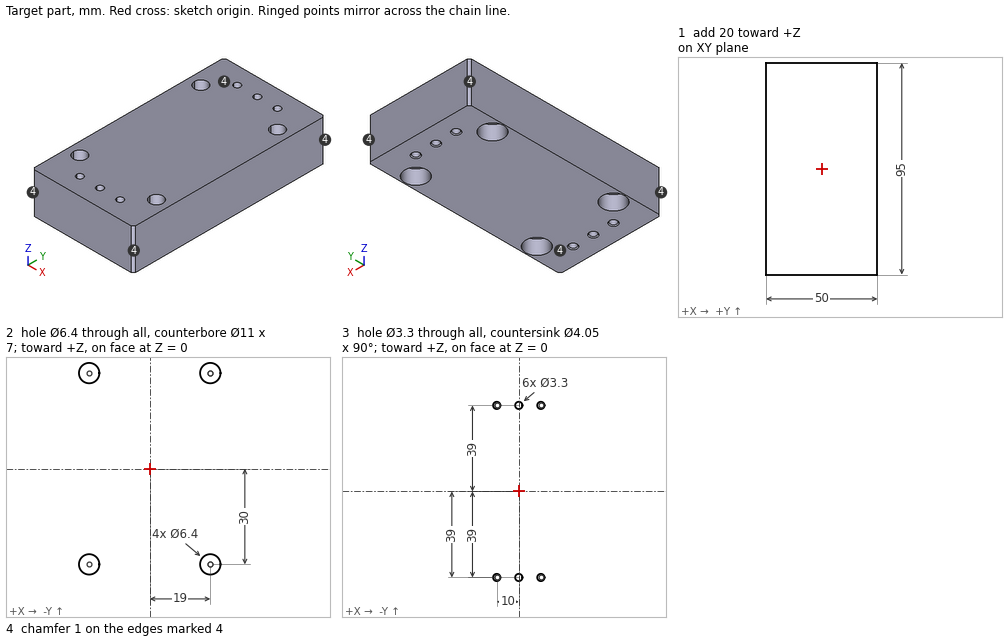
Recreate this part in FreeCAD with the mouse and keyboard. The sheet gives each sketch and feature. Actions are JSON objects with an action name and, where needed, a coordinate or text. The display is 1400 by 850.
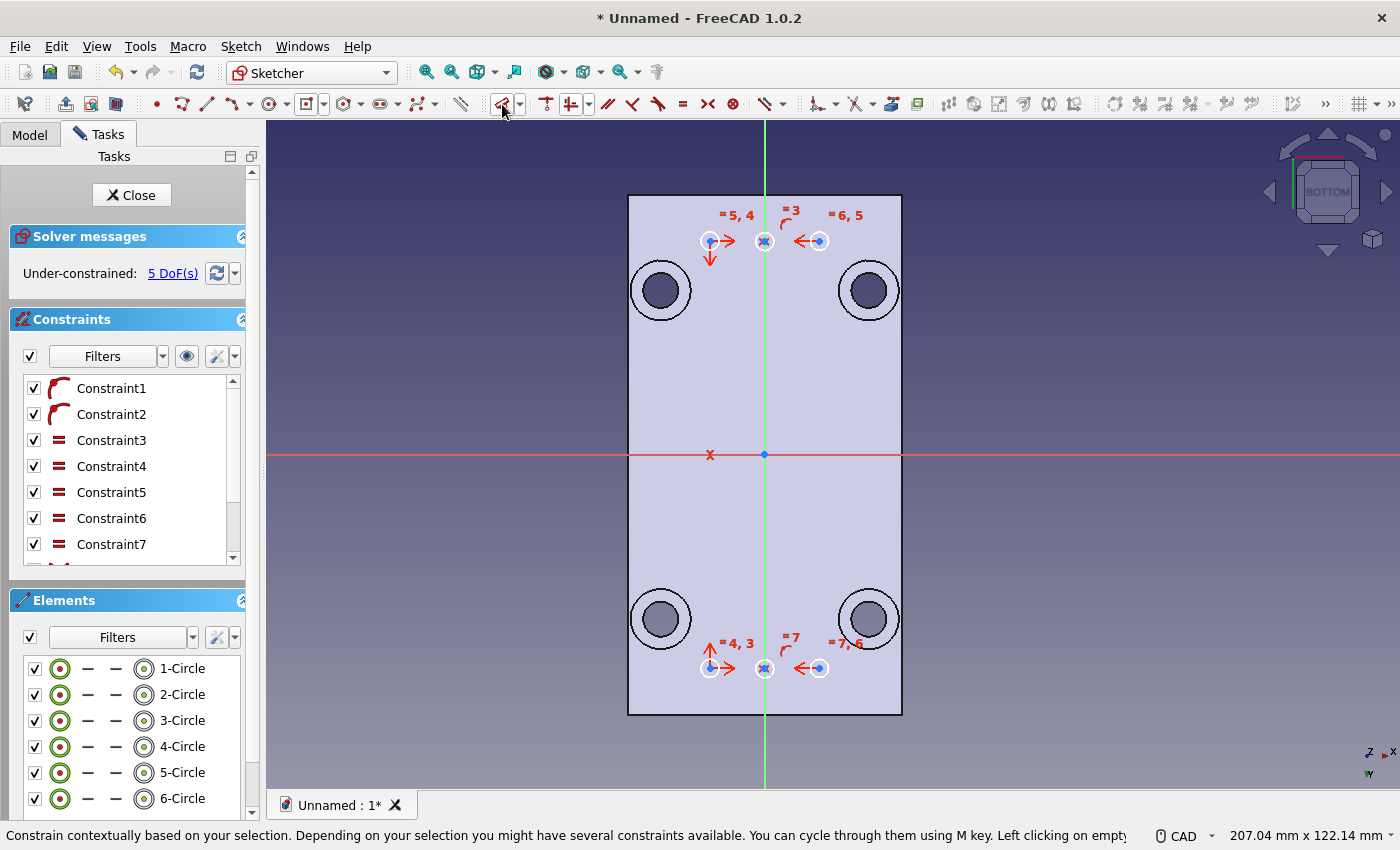
{"action": "scroll", "coordinate": [765, 233], "scroll_direction": "up", "scroll_amount": 4}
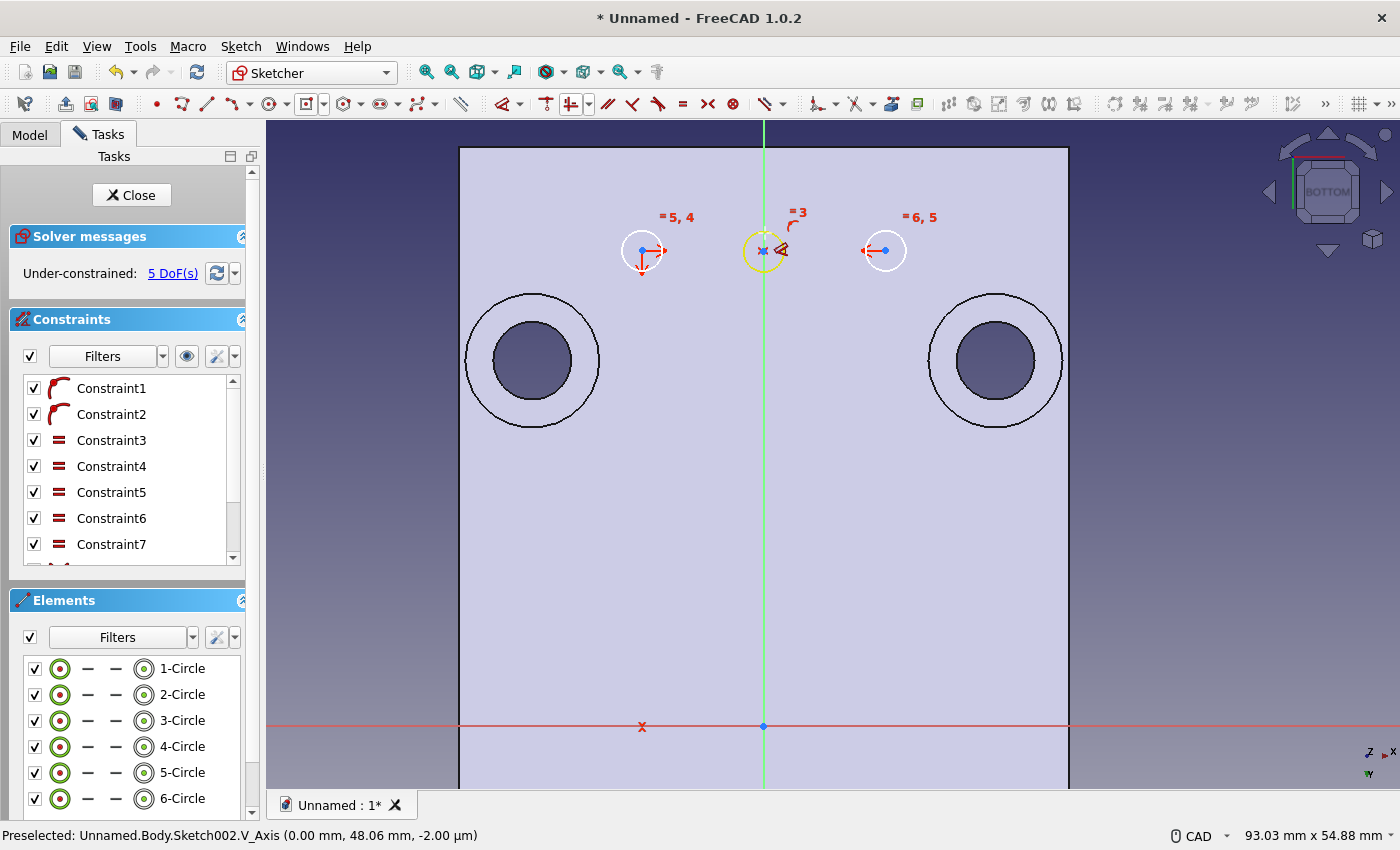
{"action": "left_click", "coordinate": [764, 232]}
{"action": "left_click", "coordinate": [789, 206]}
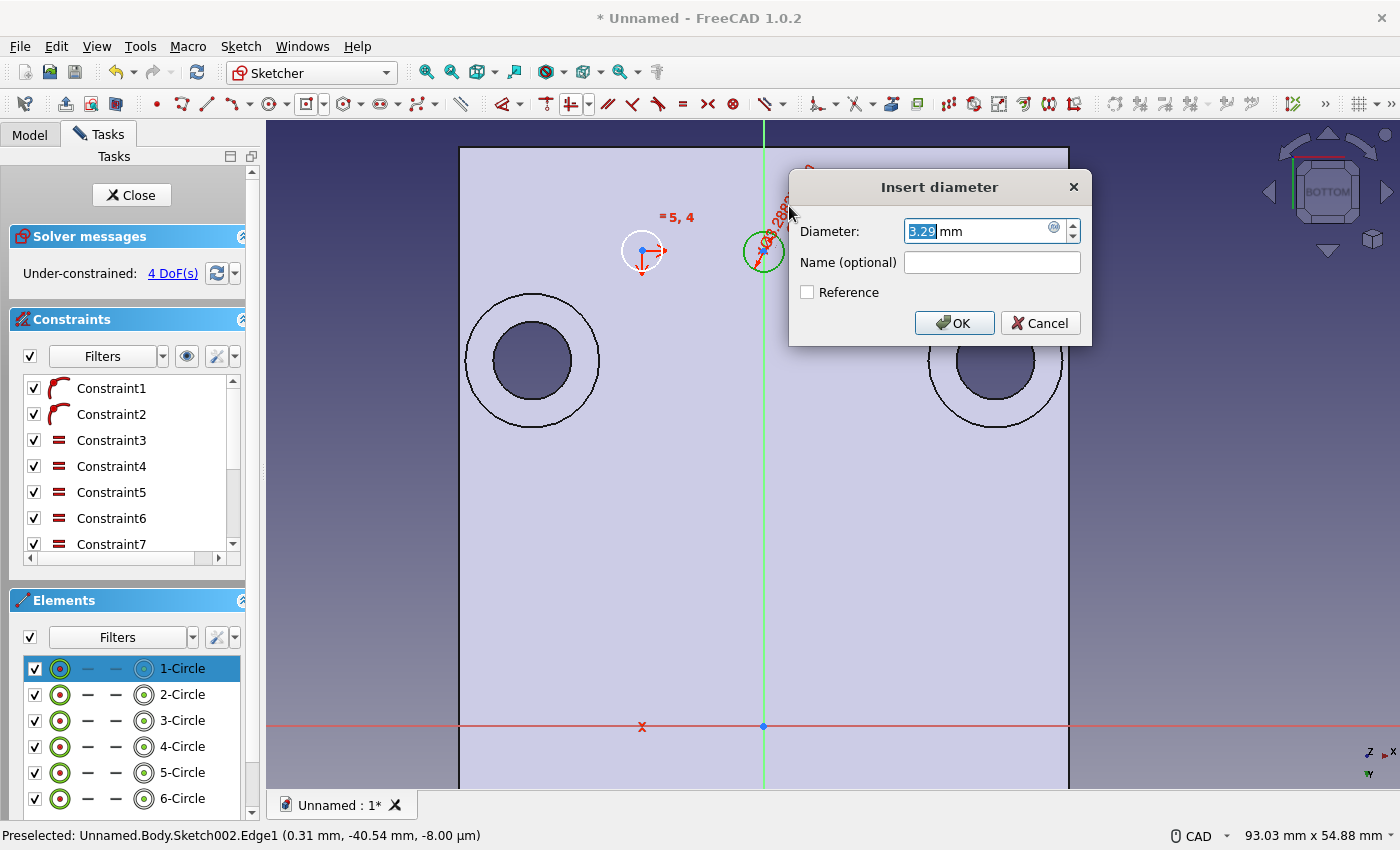
{"action": "type", "text": "3.3"}
{"action": "key", "text": "Return"}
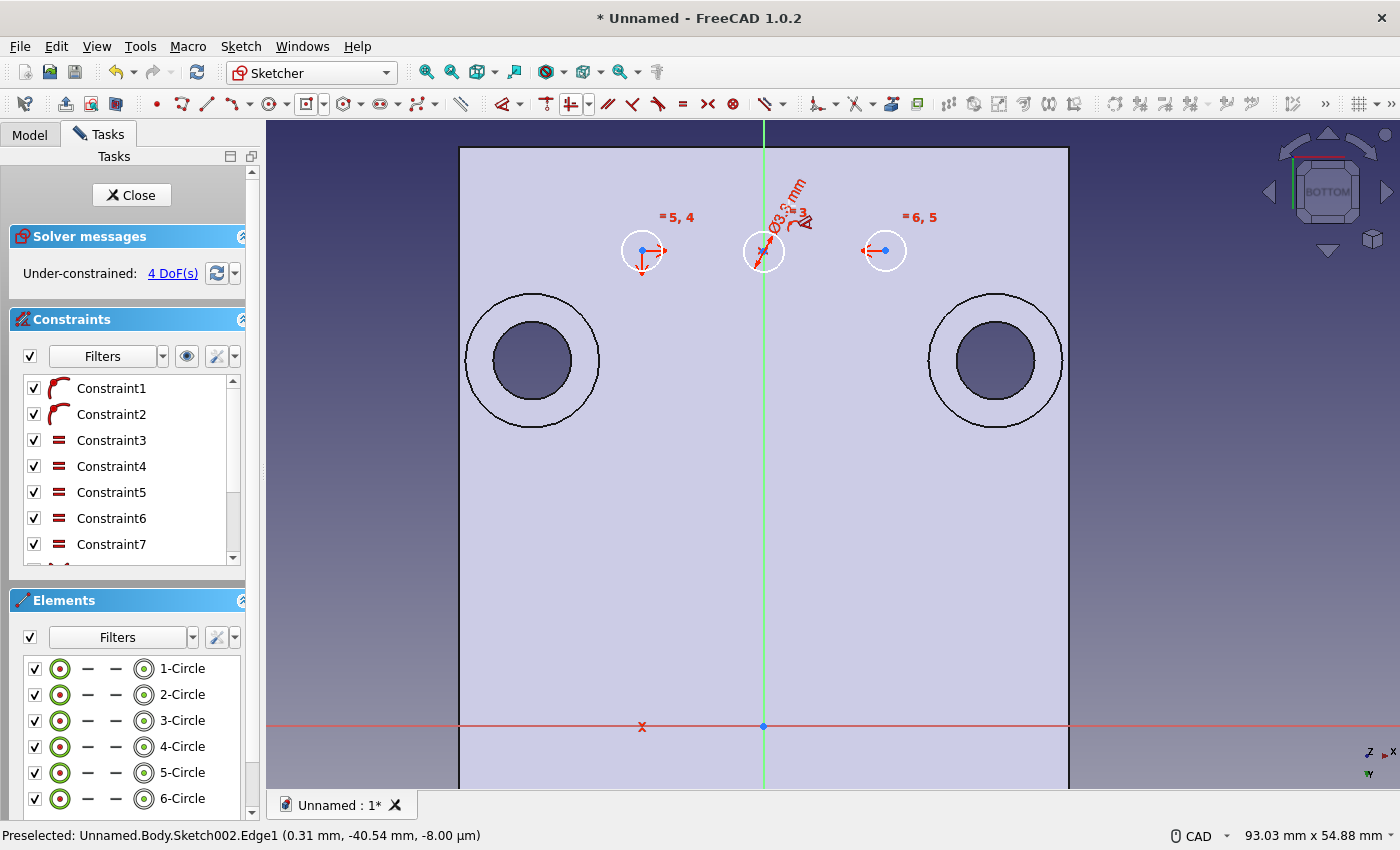
{"action": "left_click", "coordinate": [764, 252]}
{"action": "left_click", "coordinate": [798, 489]}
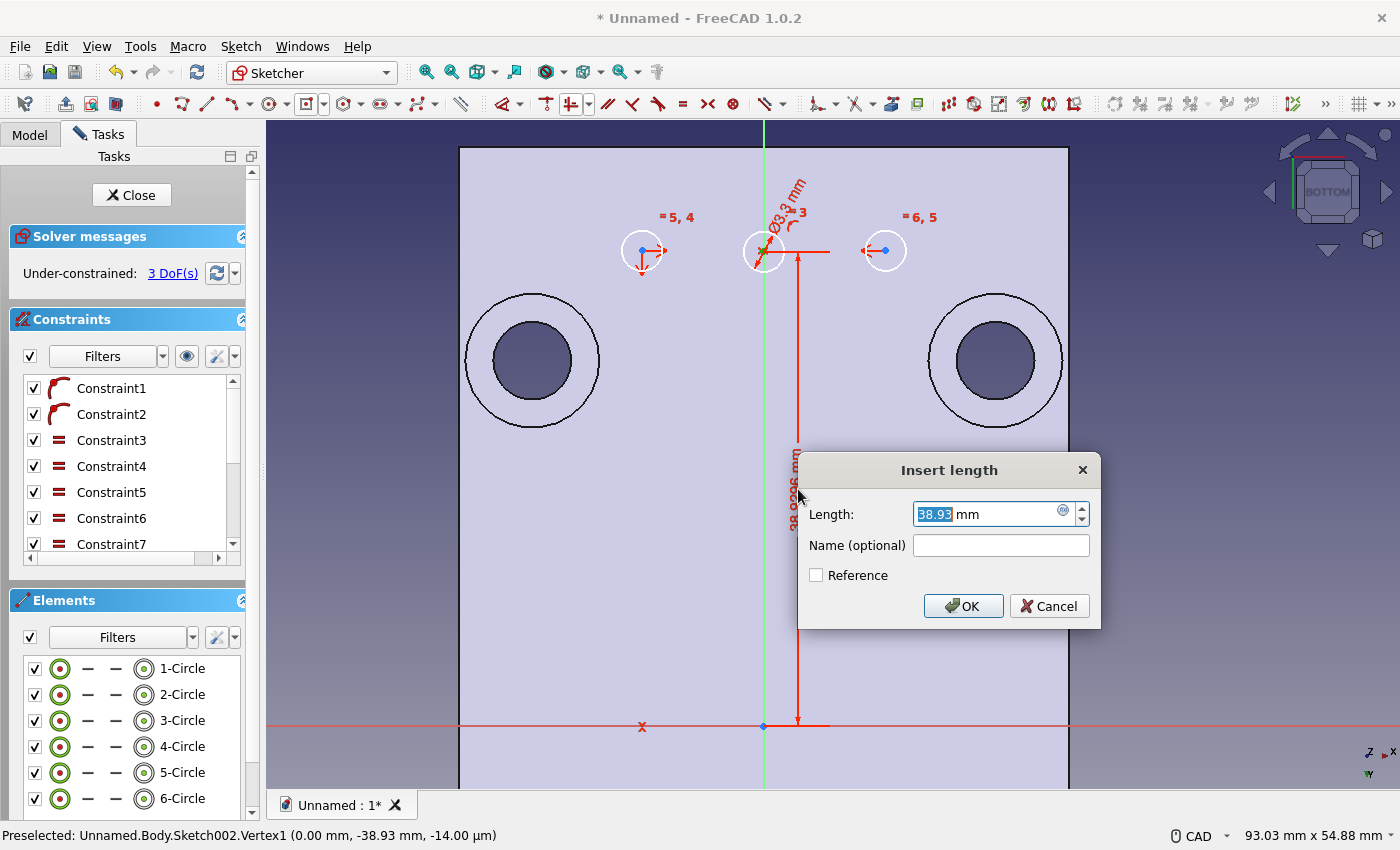
{"action": "type", "text": "39"}
{"action": "key", "text": "Return"}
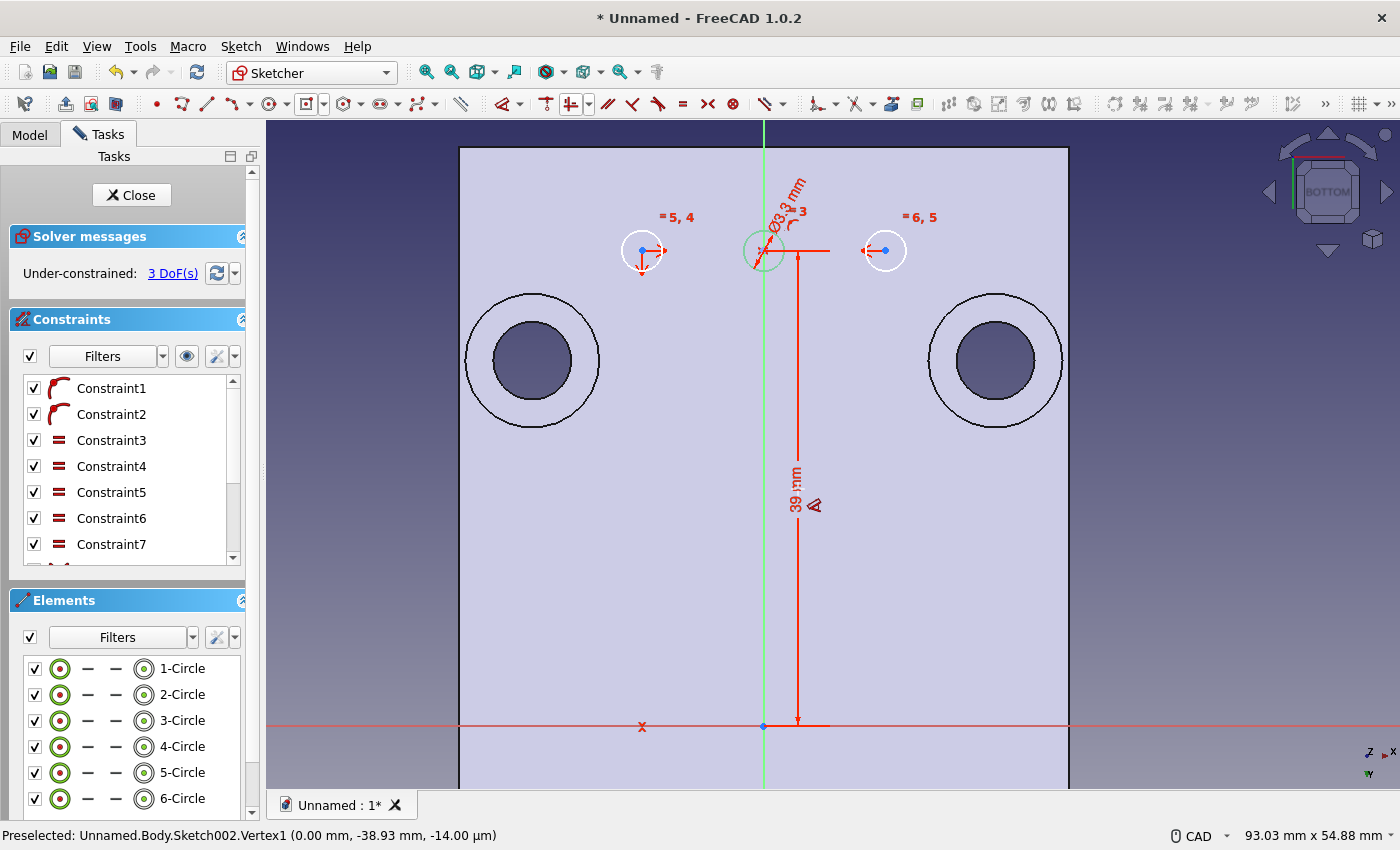
{"action": "scroll", "coordinate": [765, 233], "scroll_direction": "down", "scroll_amount": 4}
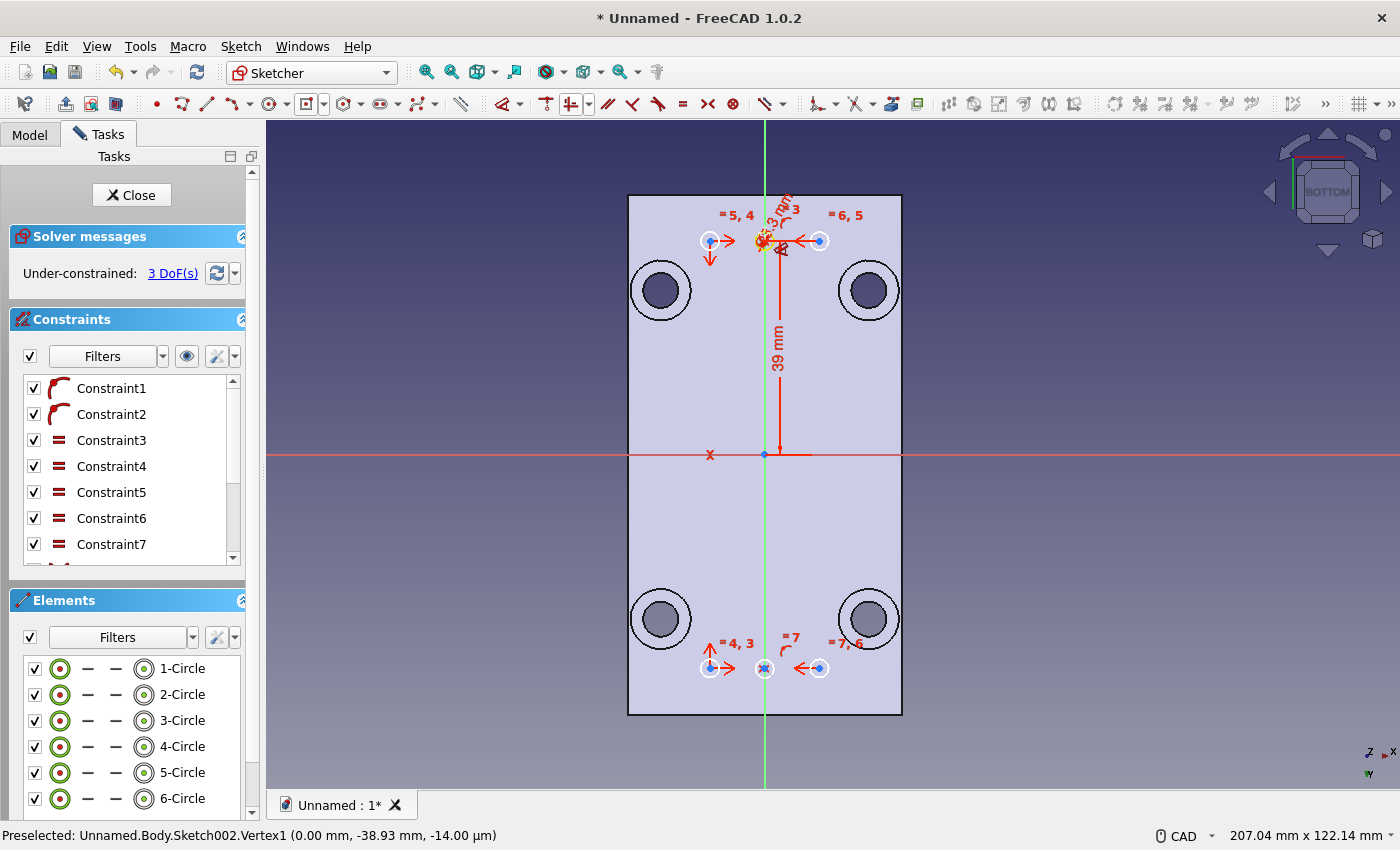
{"action": "left_click", "coordinate": [710, 668]}
{"action": "left_click", "coordinate": [737, 702]}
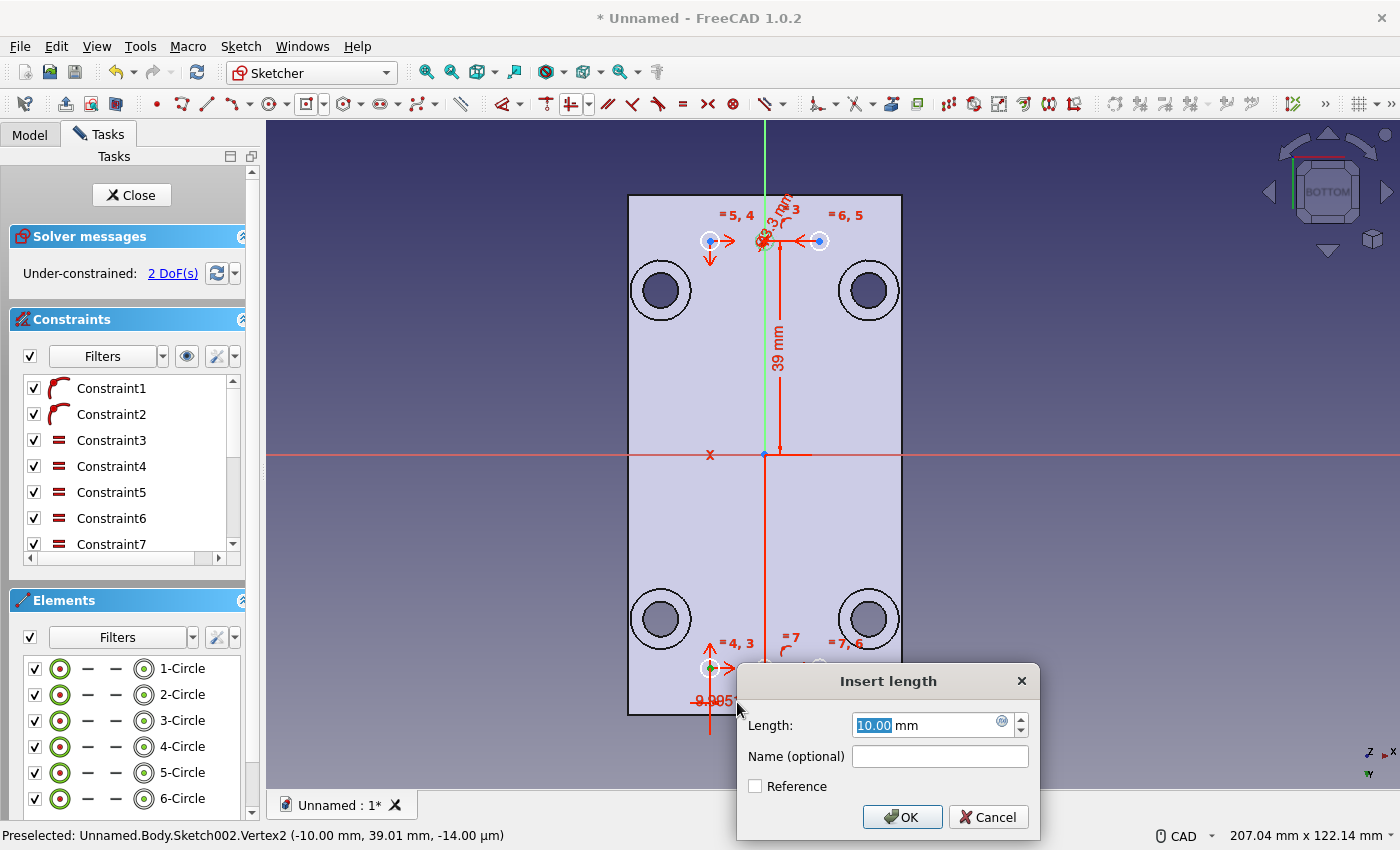
{"action": "type", "text": "10"}
{"action": "key", "text": "Return"}